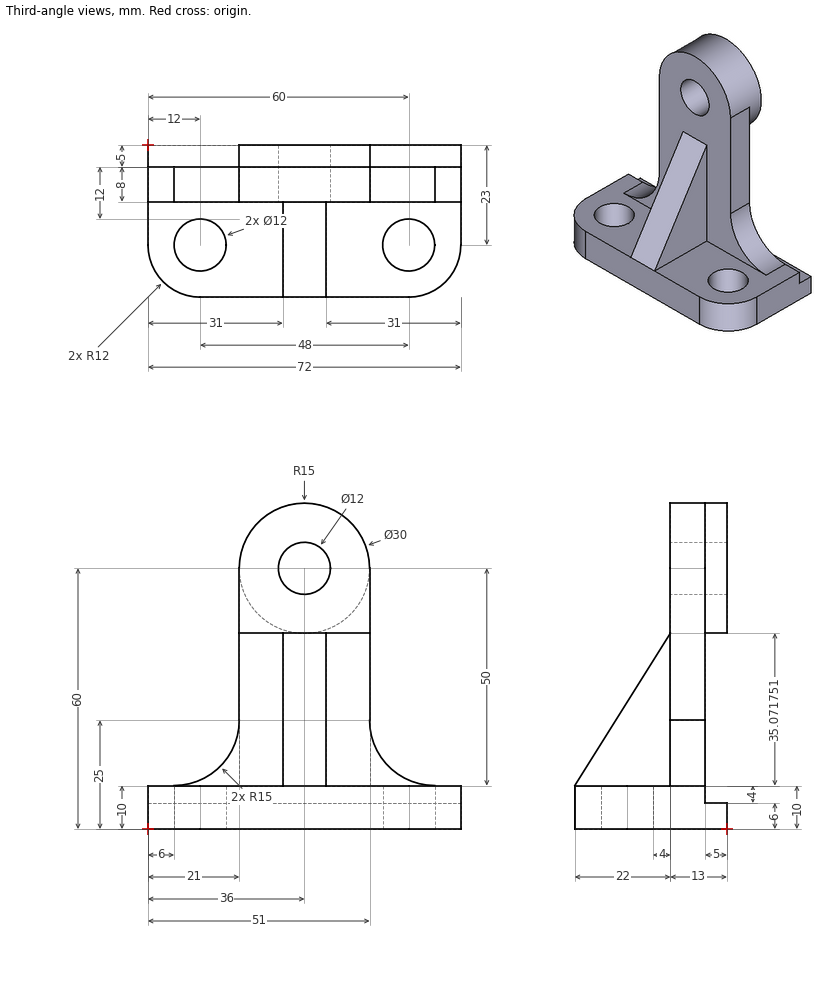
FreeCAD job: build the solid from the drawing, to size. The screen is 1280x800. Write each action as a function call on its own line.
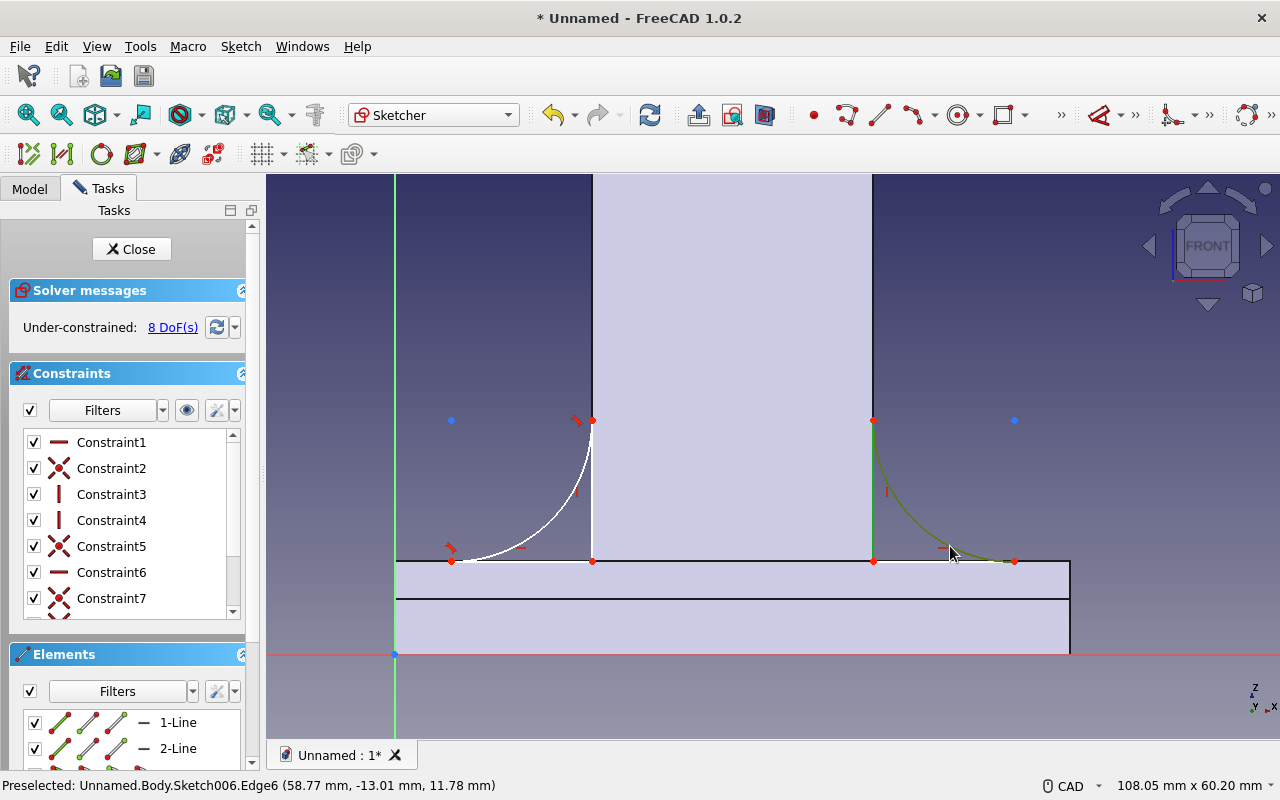
key(t)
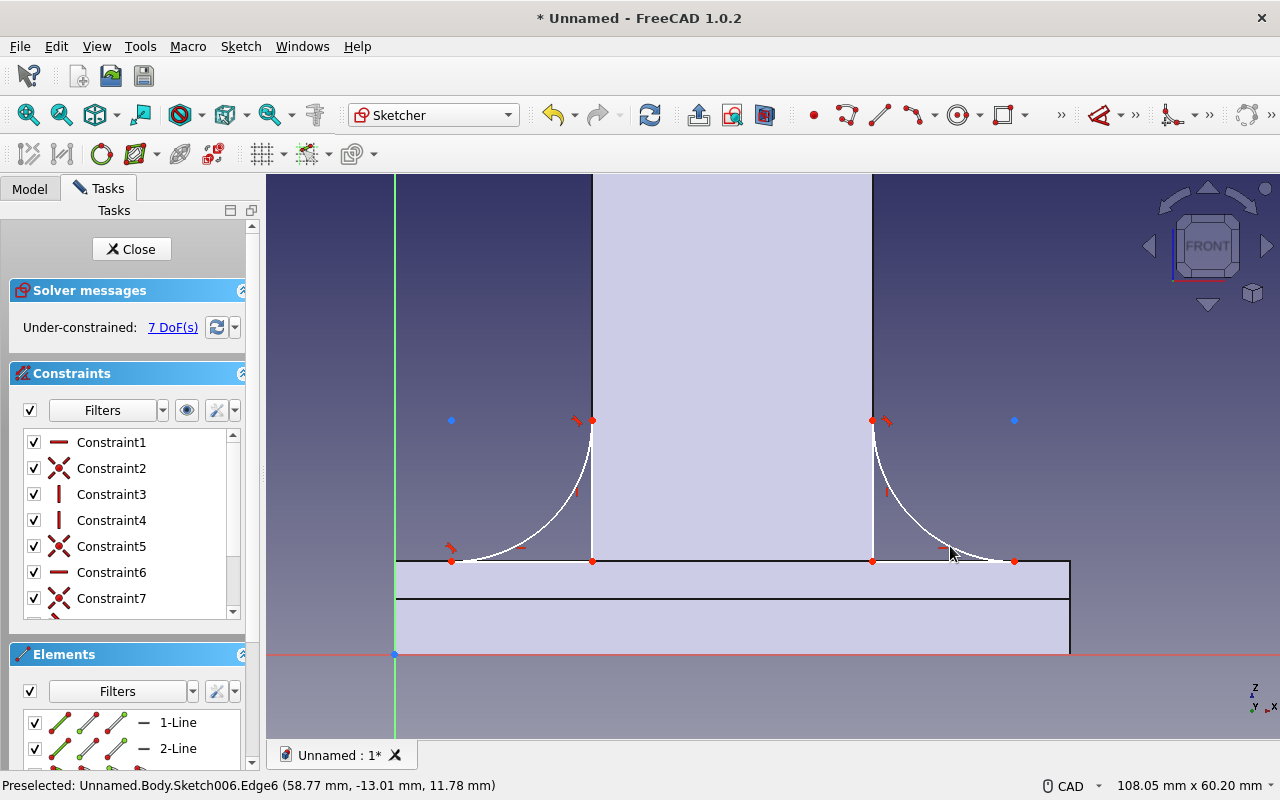
click(915, 562)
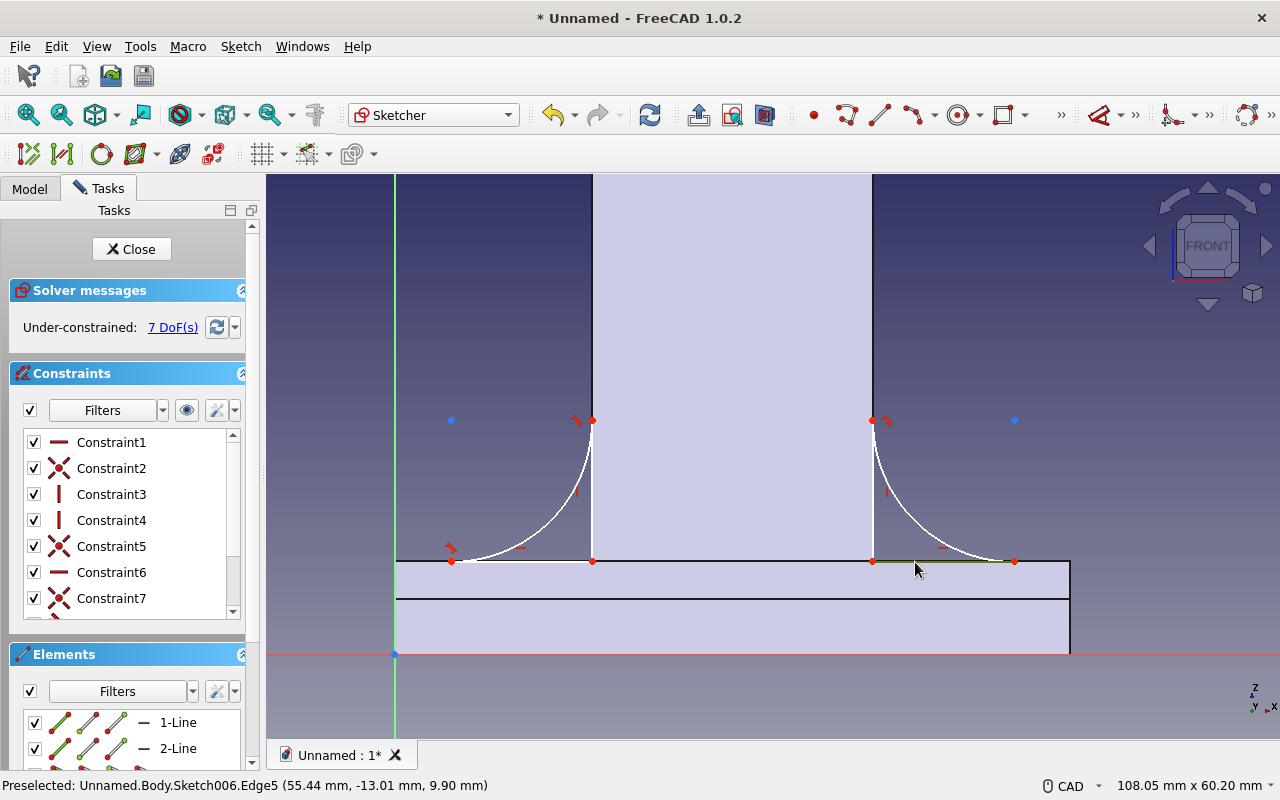
click(888, 484)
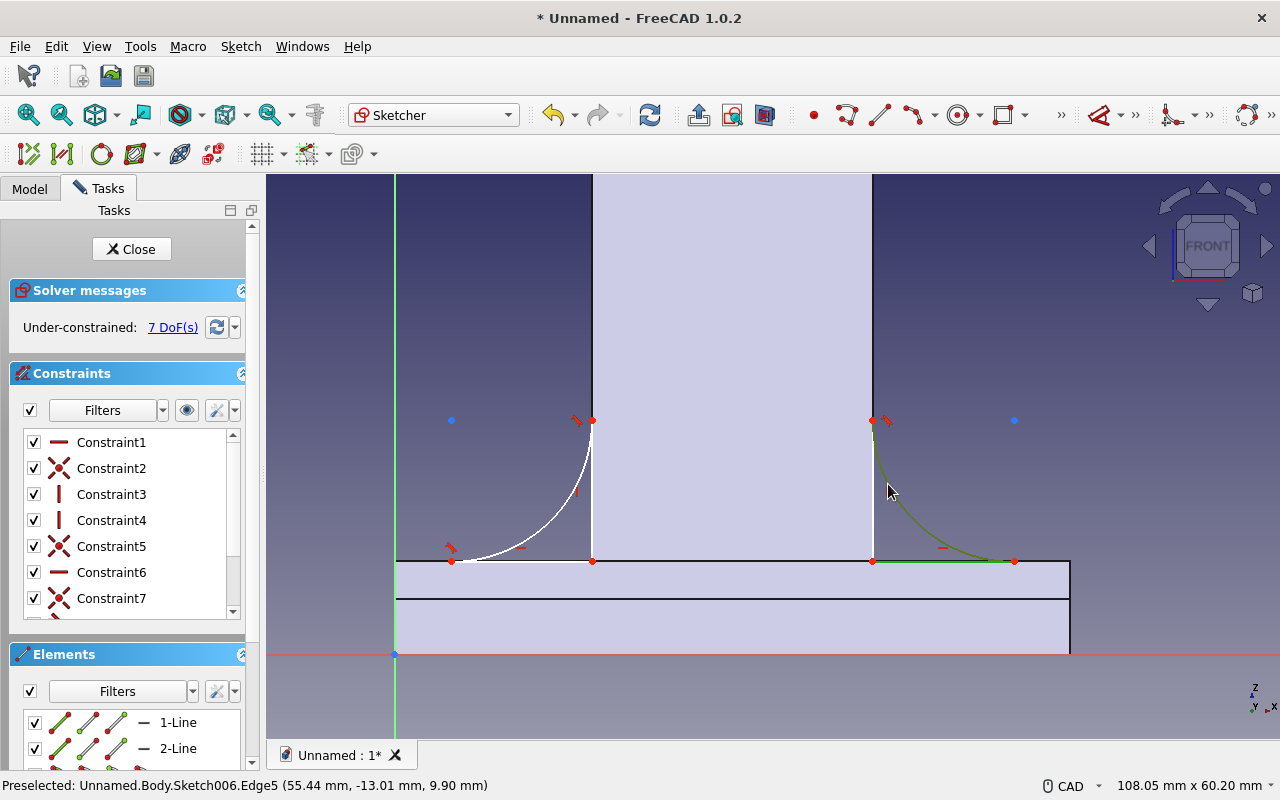
key(t)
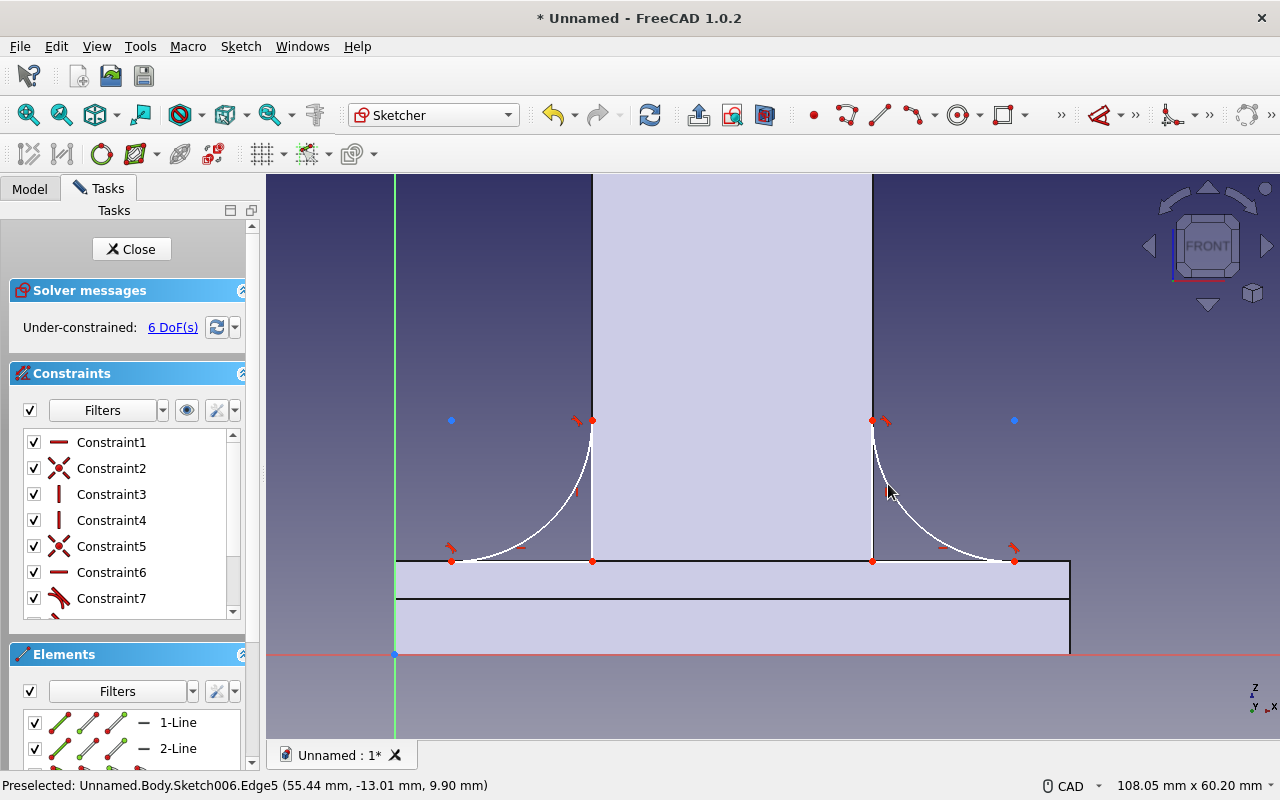
click(515, 547)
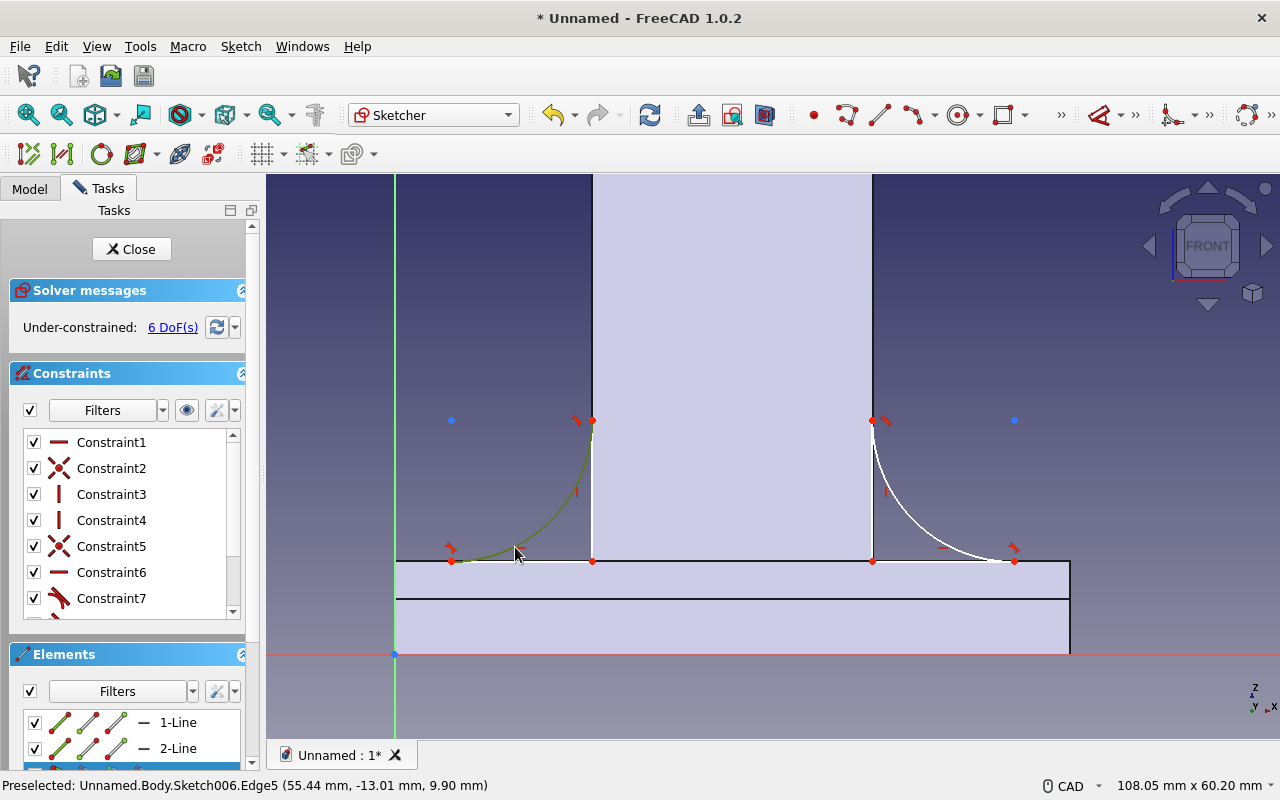
click(950, 547)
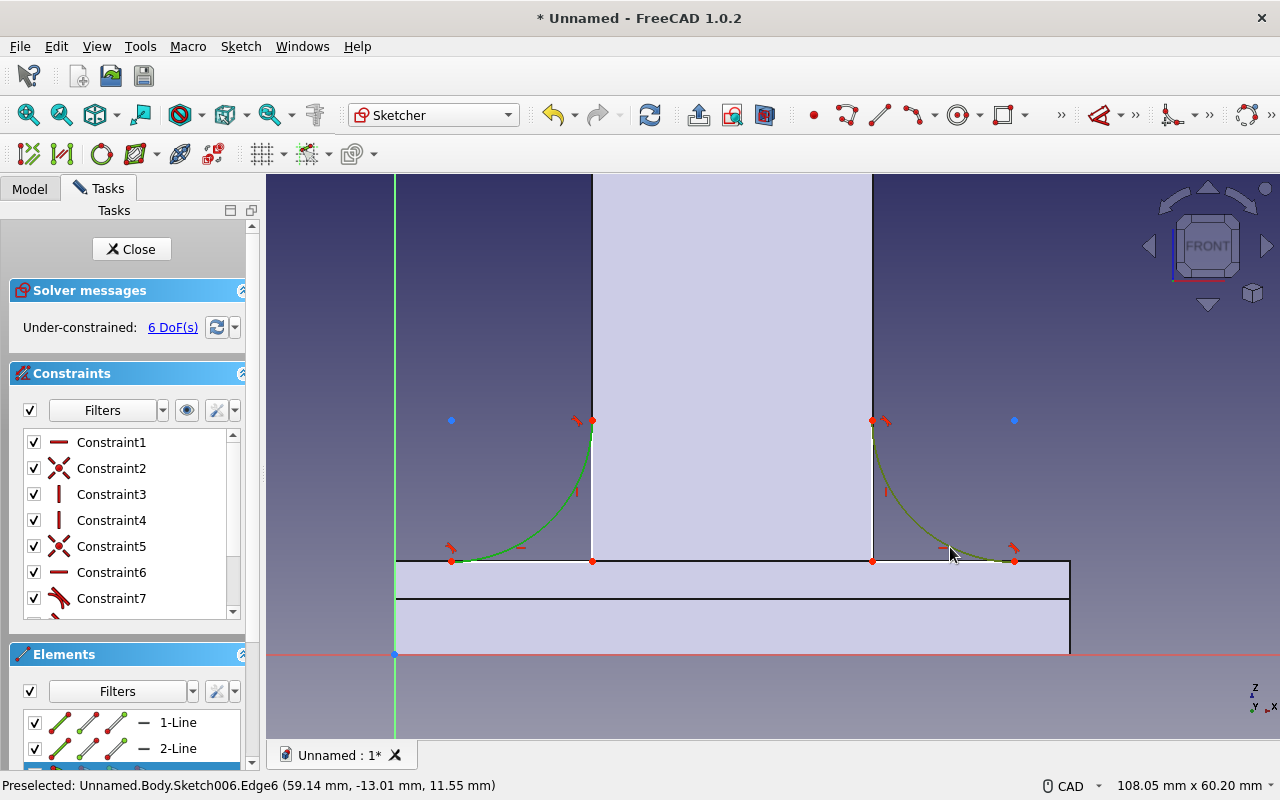
key(e)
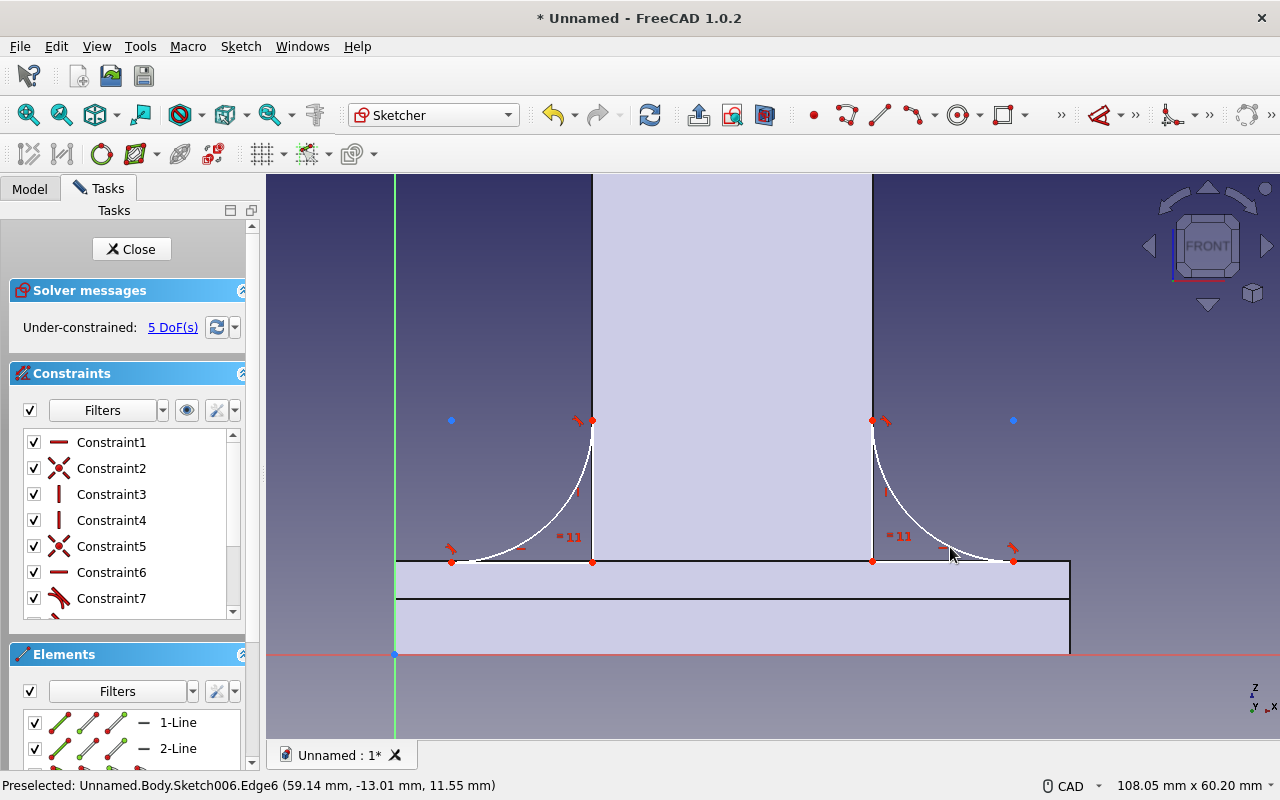
click(1098, 116)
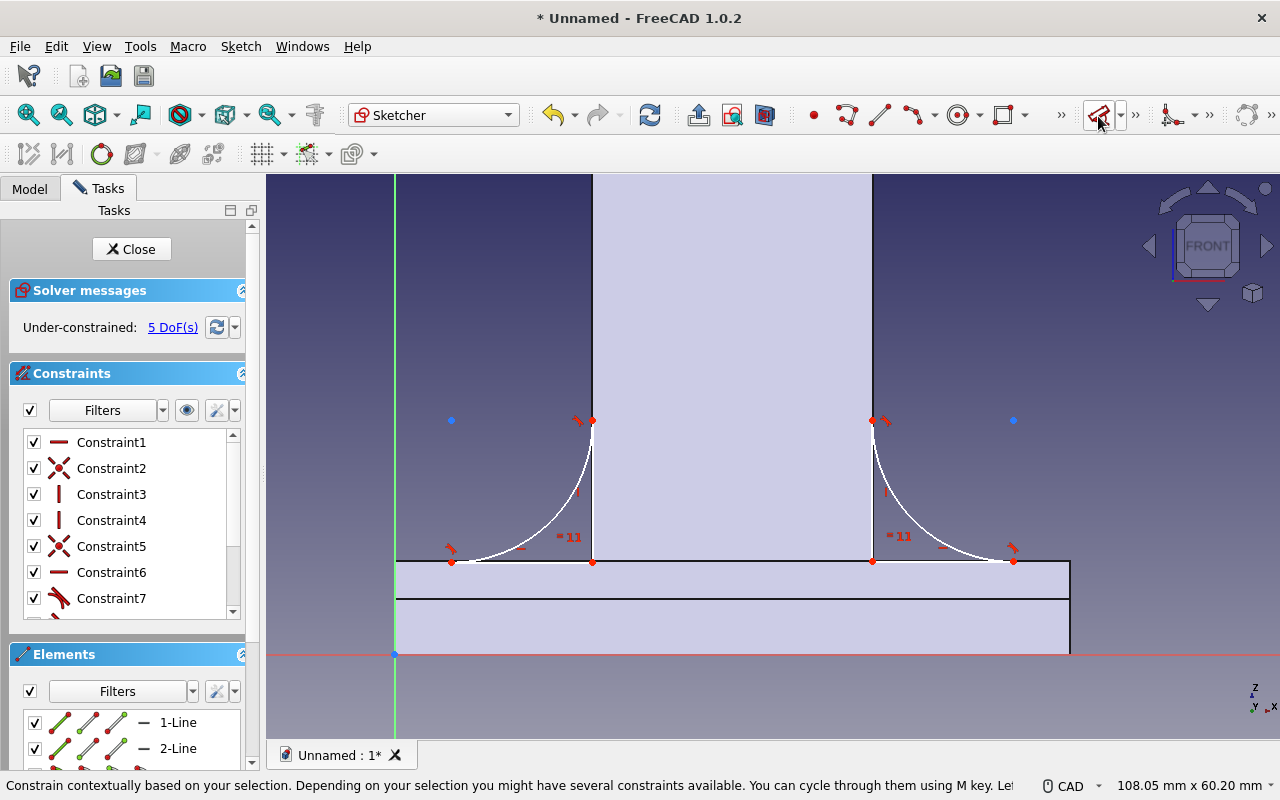
click(515, 547)
click(446, 594)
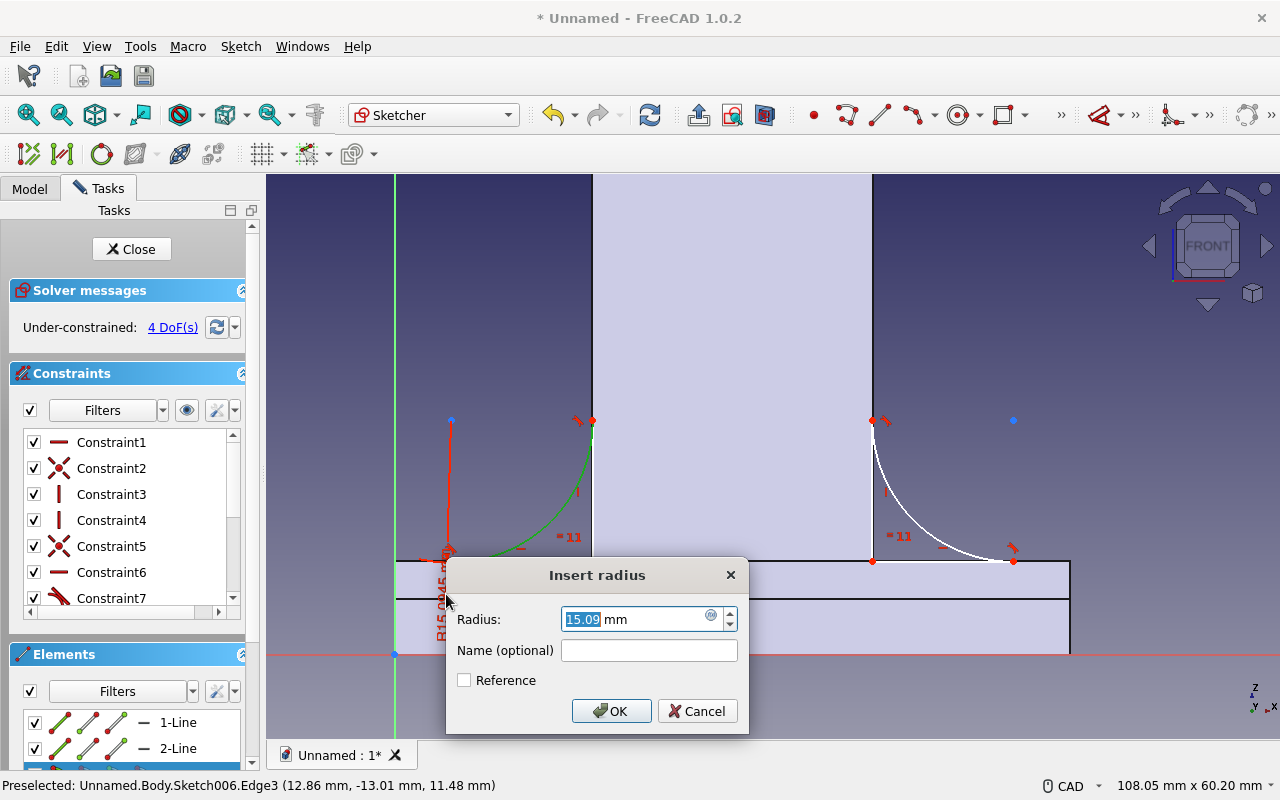
text(15)
key(Return)